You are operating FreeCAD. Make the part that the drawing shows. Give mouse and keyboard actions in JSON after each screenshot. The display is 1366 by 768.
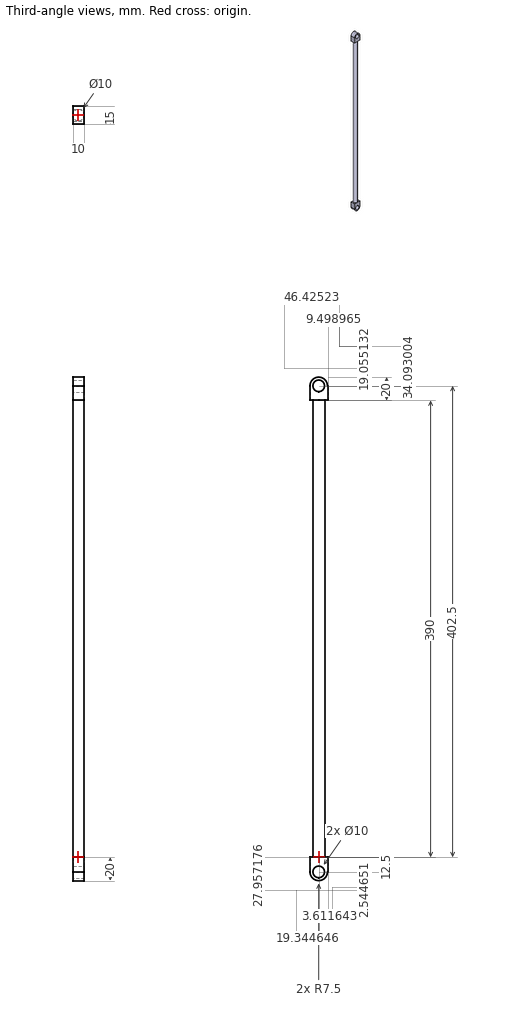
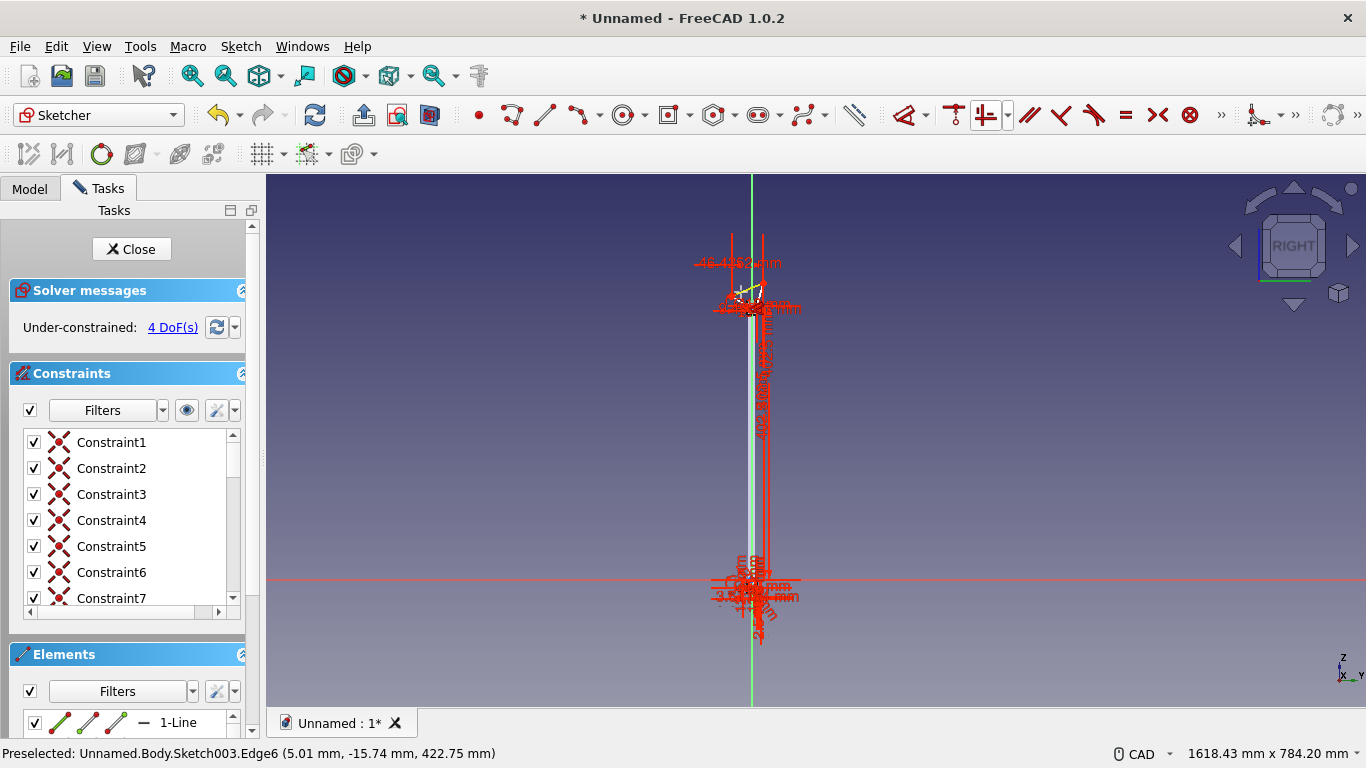
{"action": "scroll", "coordinate": [739, 599], "scroll_direction": "up", "scroll_amount": 6}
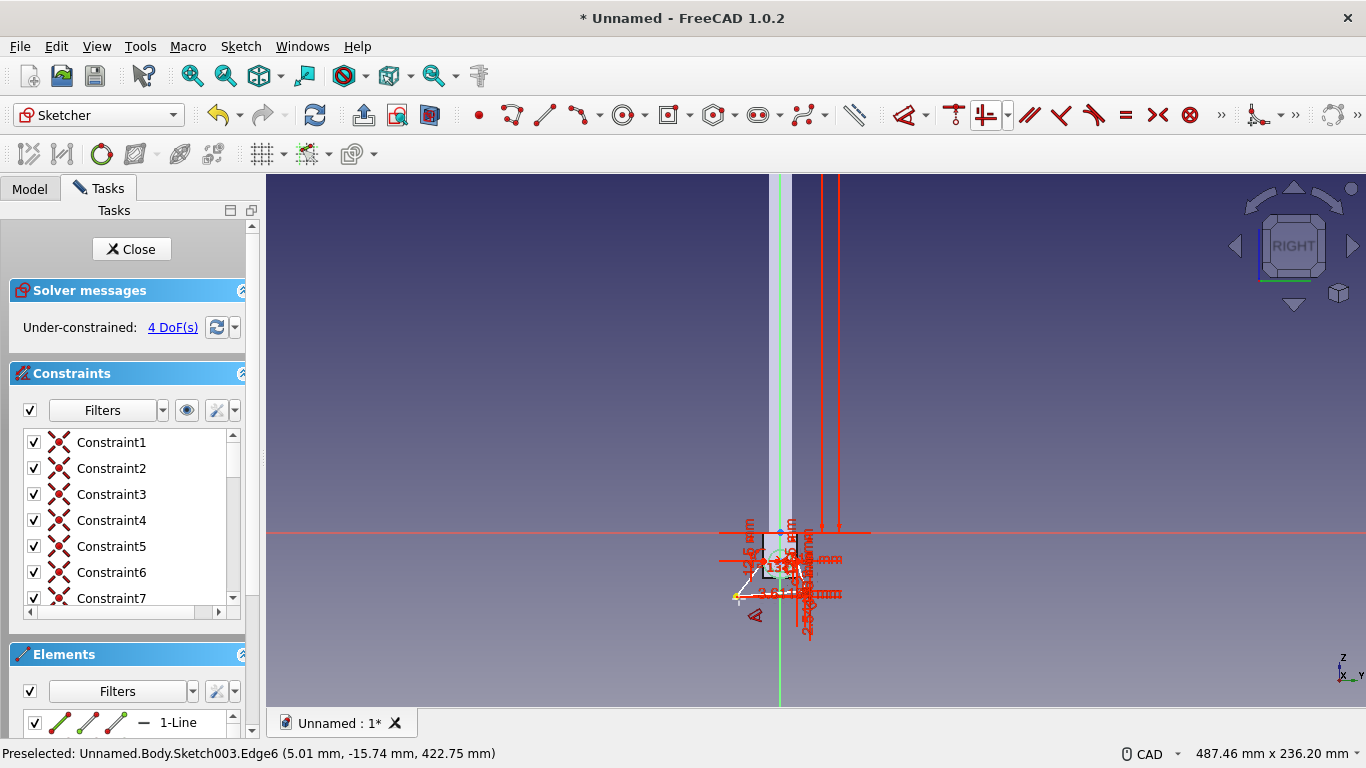
{"action": "left_click", "coordinate": [736, 597]}
{"action": "left_click", "coordinate": [758, 631]}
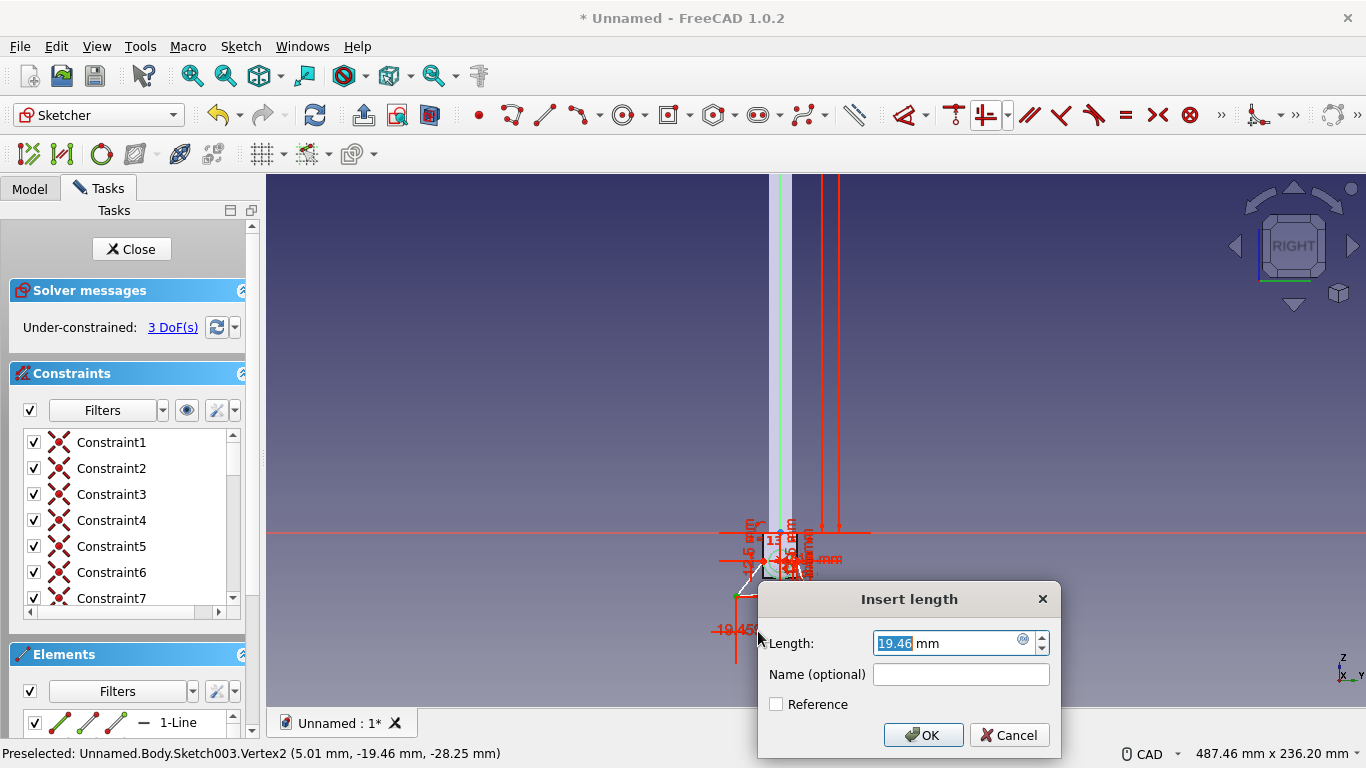
{"action": "type", "text": "19.344646"}
{"action": "key", "text": "Return"}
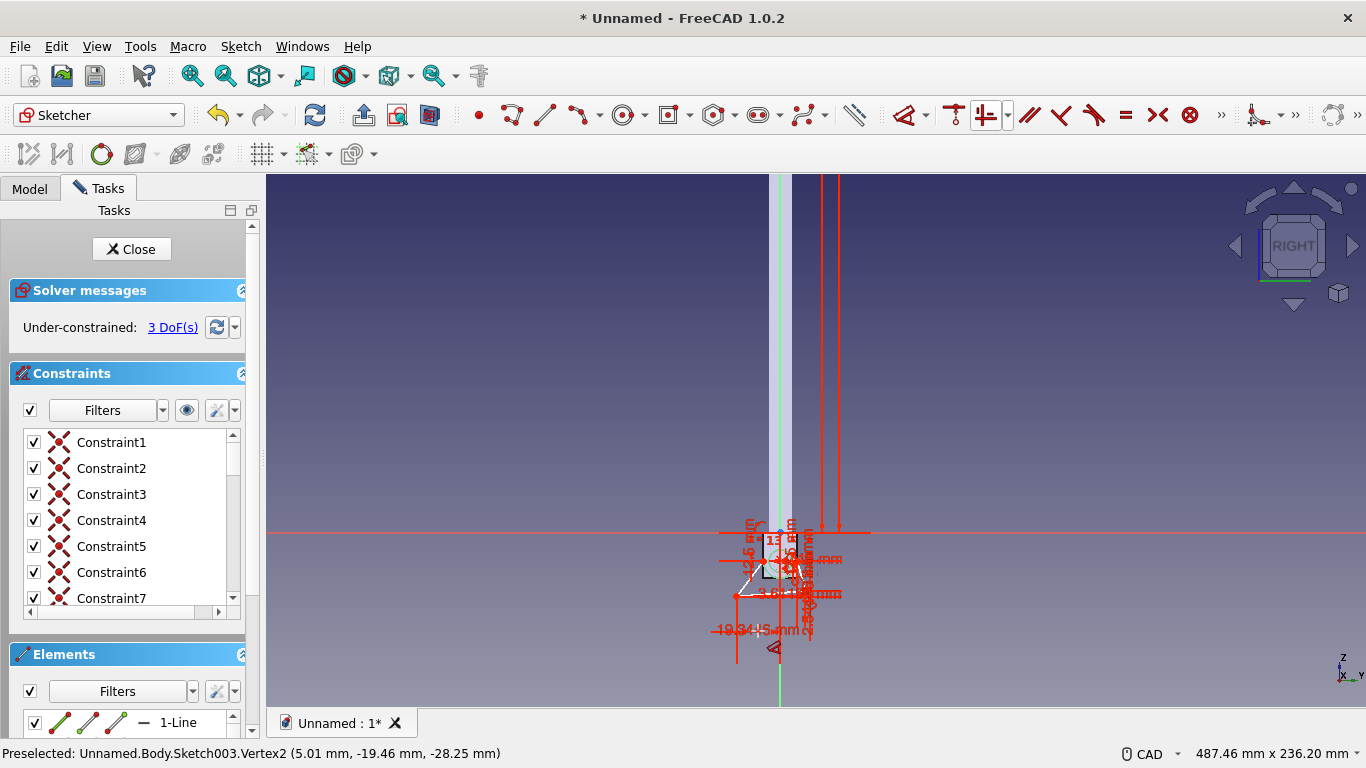
{"action": "left_click", "coordinate": [737, 597]}
{"action": "left_click", "coordinate": [703, 580]}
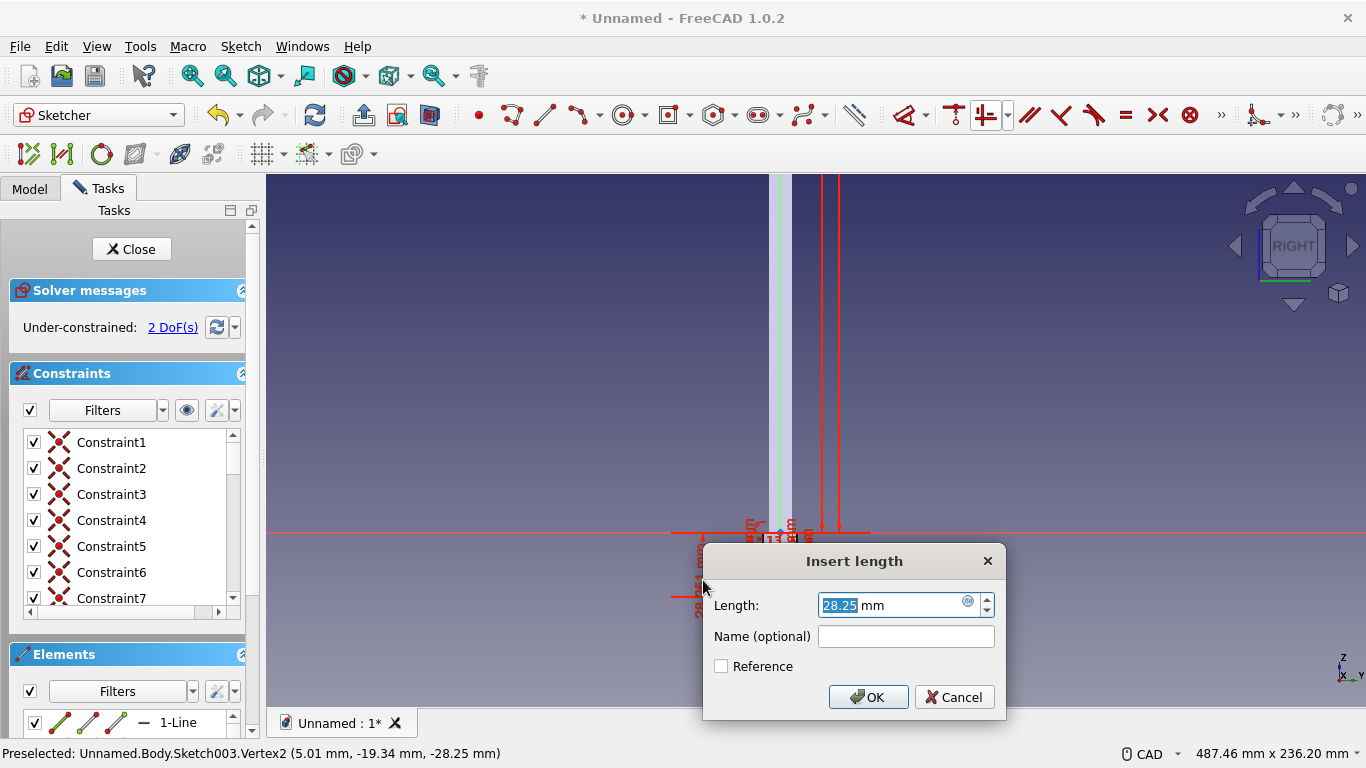
{"action": "type", "text": "27.957176"}
{"action": "key", "text": "Return"}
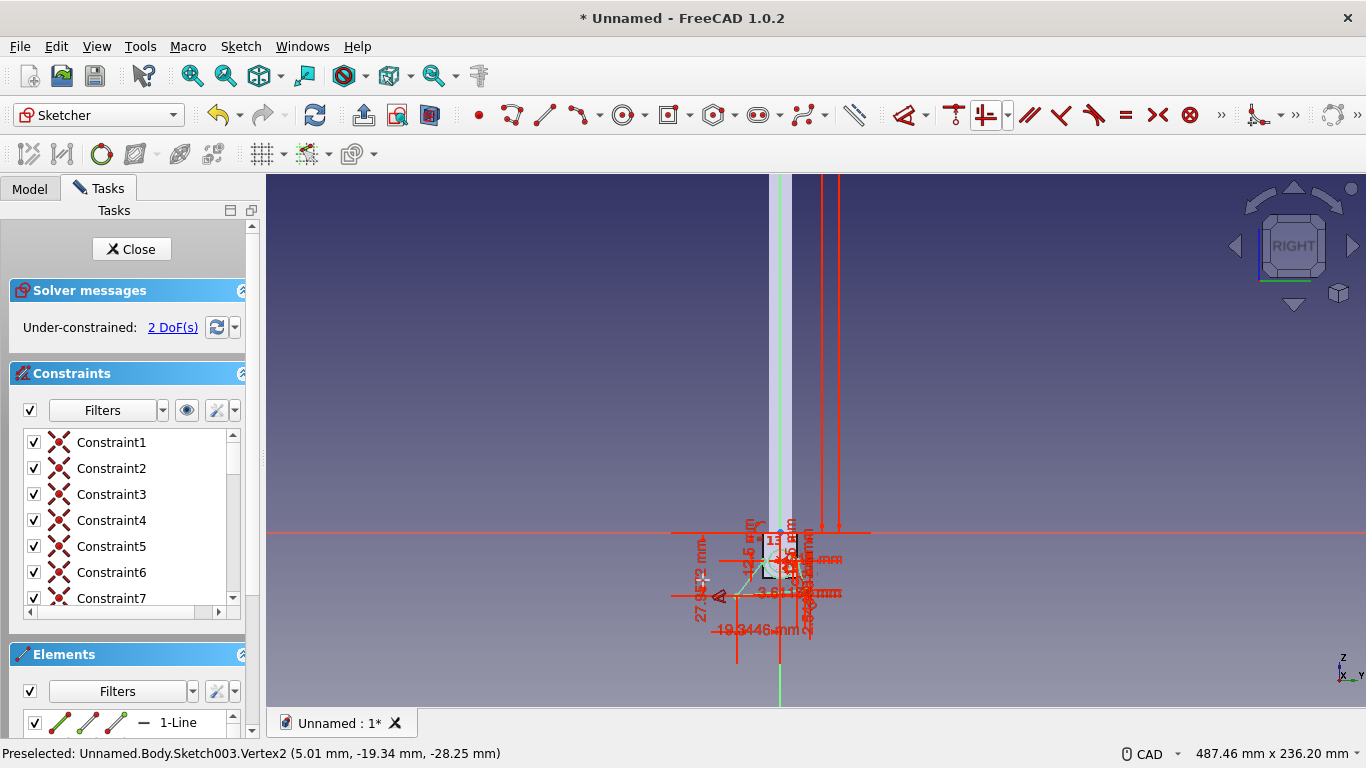
{"action": "scroll", "coordinate": [739, 599], "scroll_direction": "down", "scroll_amount": 6}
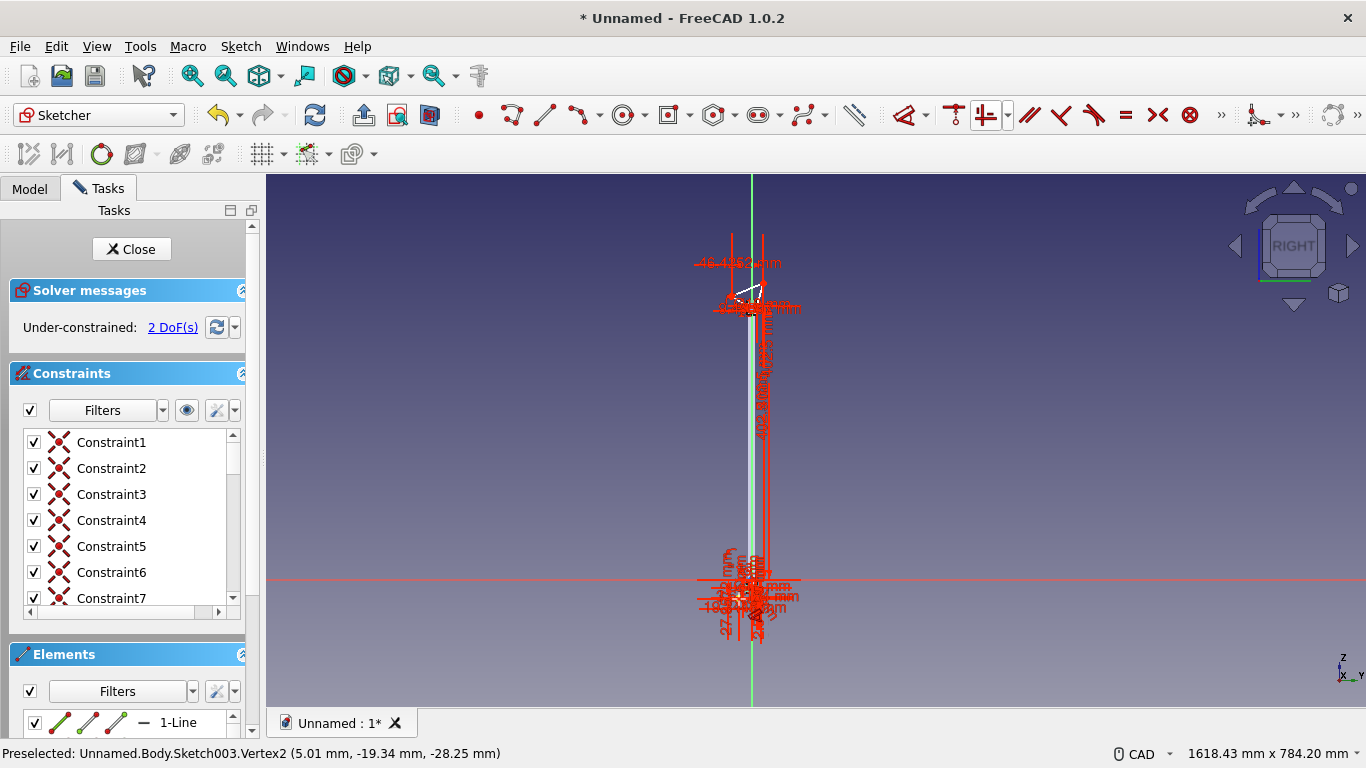
{"action": "scroll", "coordinate": [759, 299], "scroll_direction": "up", "scroll_amount": 6}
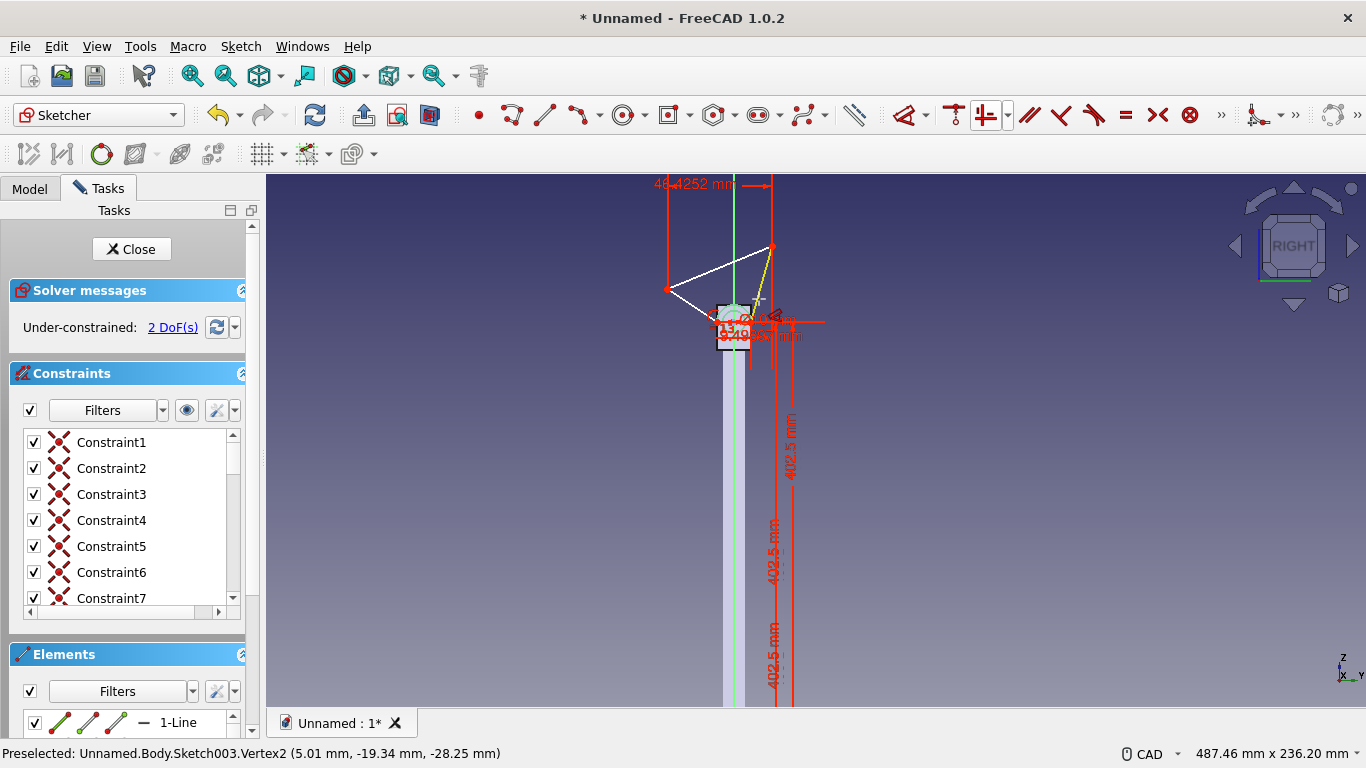
{"action": "left_click", "coordinate": [757, 299]}
{"action": "left_click", "coordinate": [806, 284]}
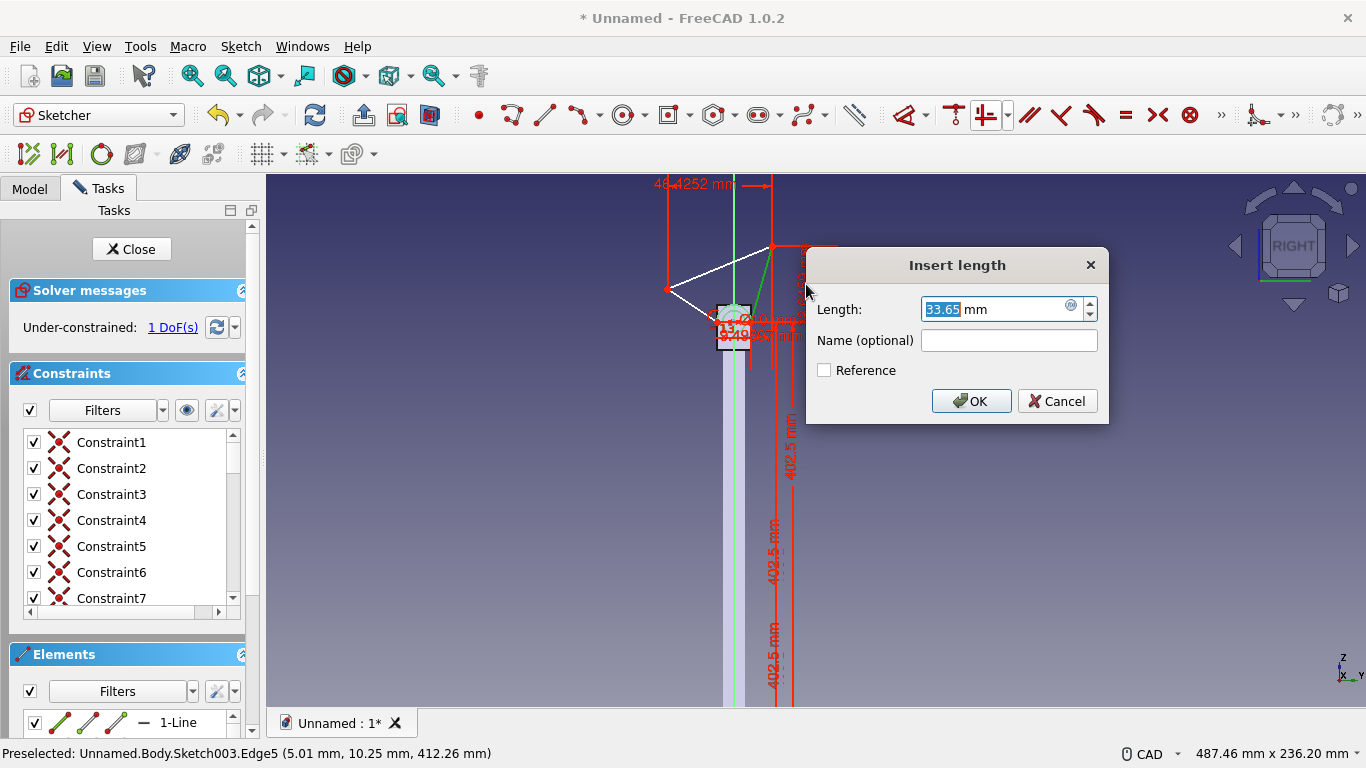
{"action": "type", "text": "34.093004"}
{"action": "key", "text": "Return"}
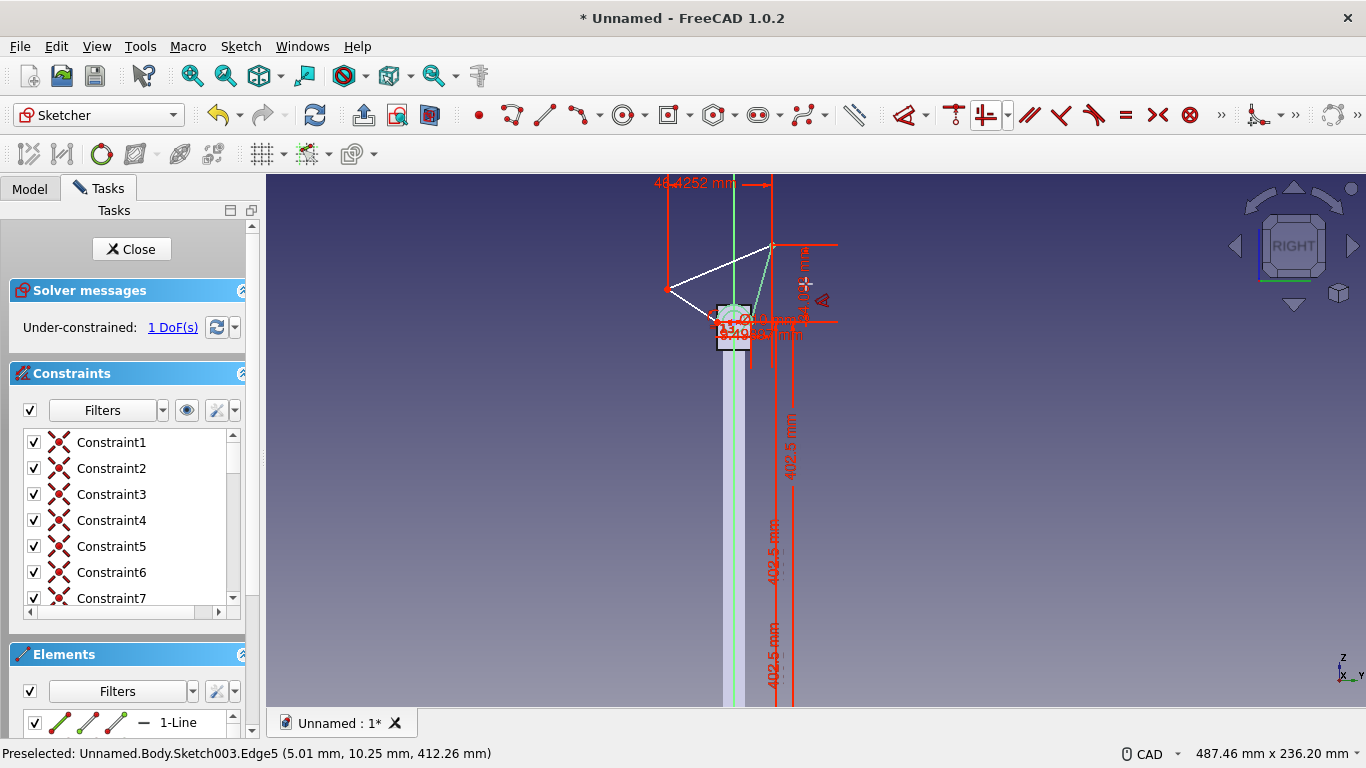
{"action": "left_click", "coordinate": [699, 276]}
{"action": "left_click", "coordinate": [806, 257]}